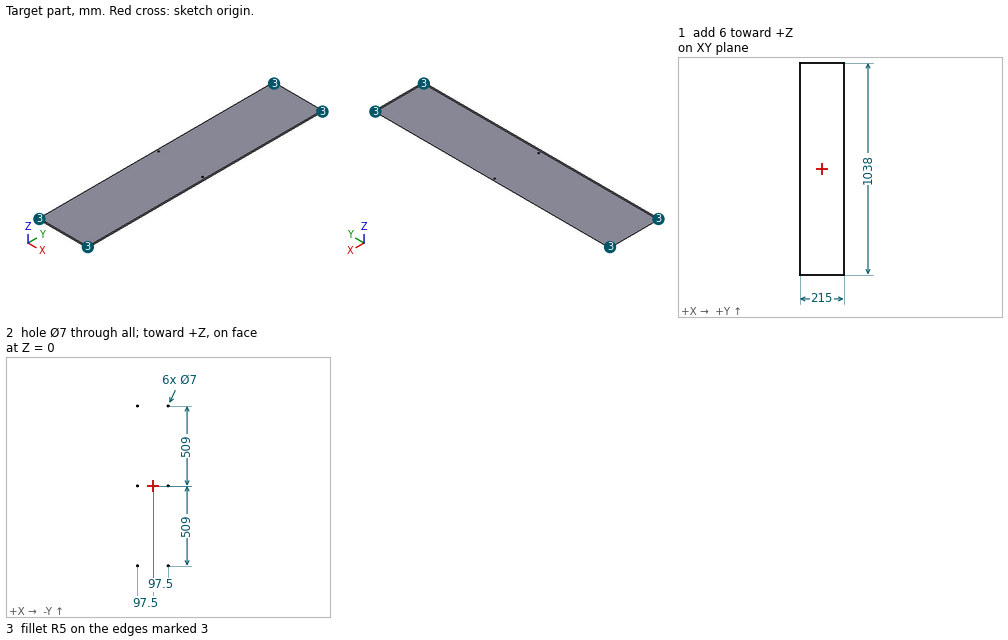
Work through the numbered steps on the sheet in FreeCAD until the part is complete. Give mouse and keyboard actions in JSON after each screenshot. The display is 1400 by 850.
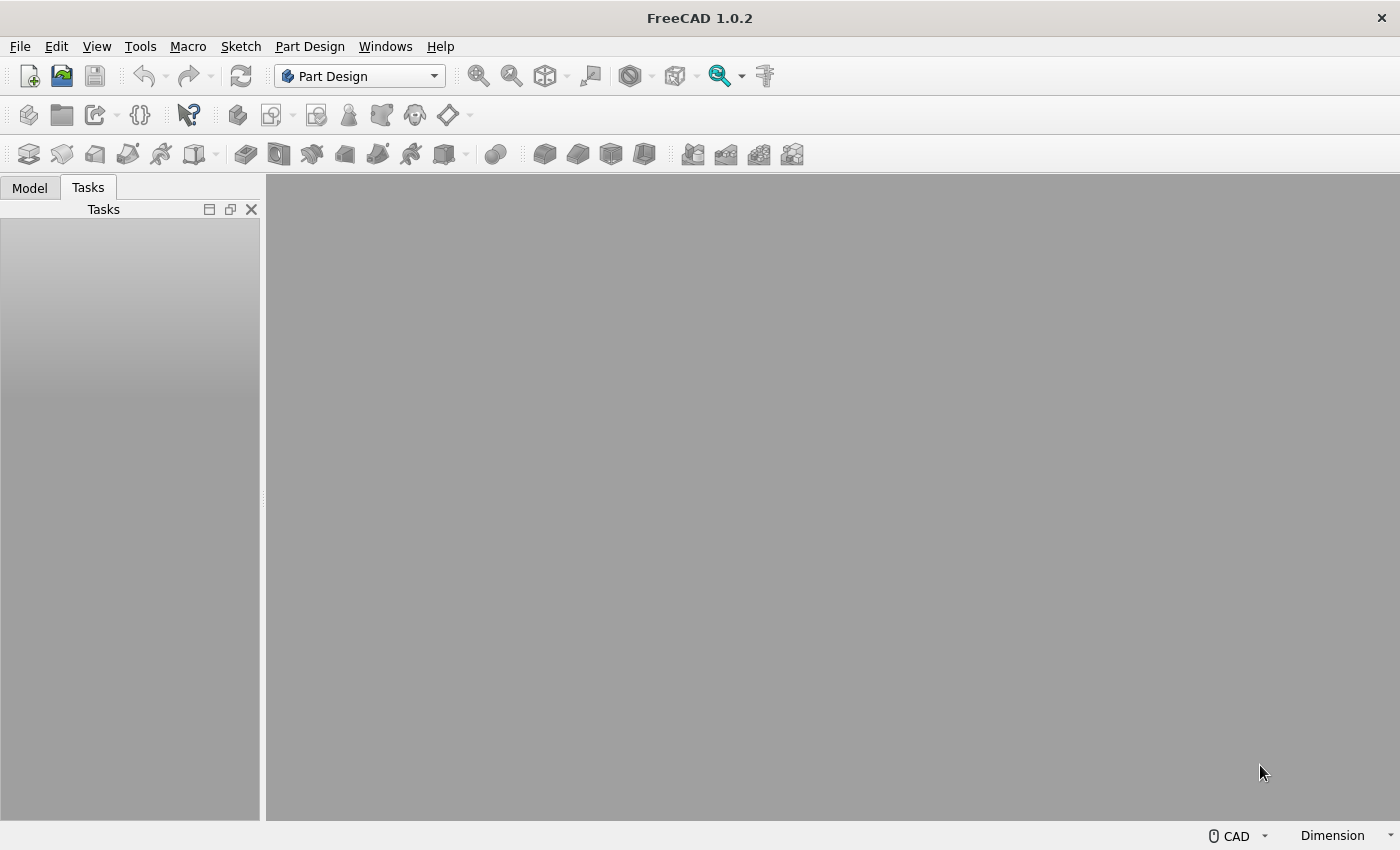
{"action": "left_click", "coordinate": [29, 76]}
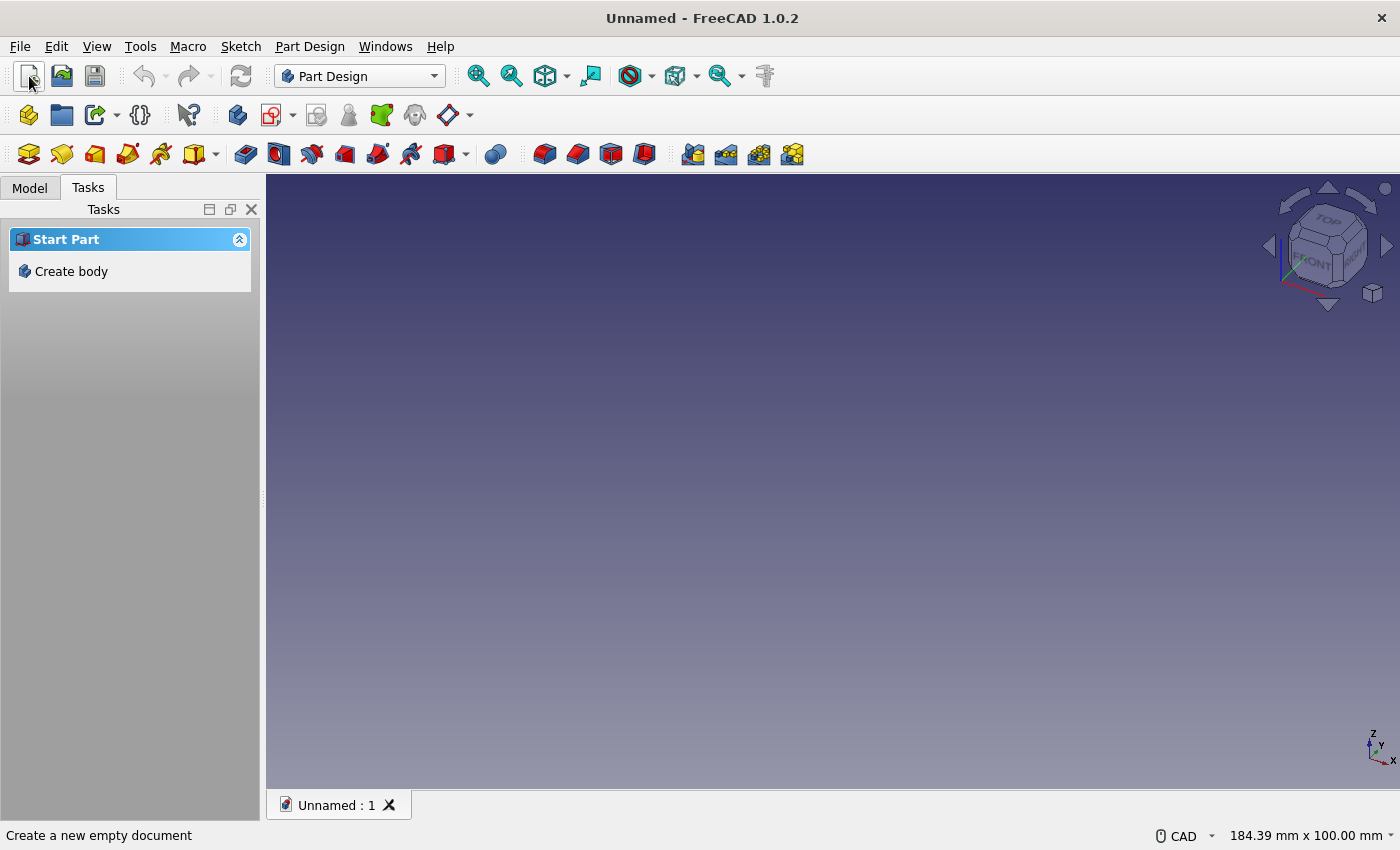
{"action": "left_click", "coordinate": [270, 116]}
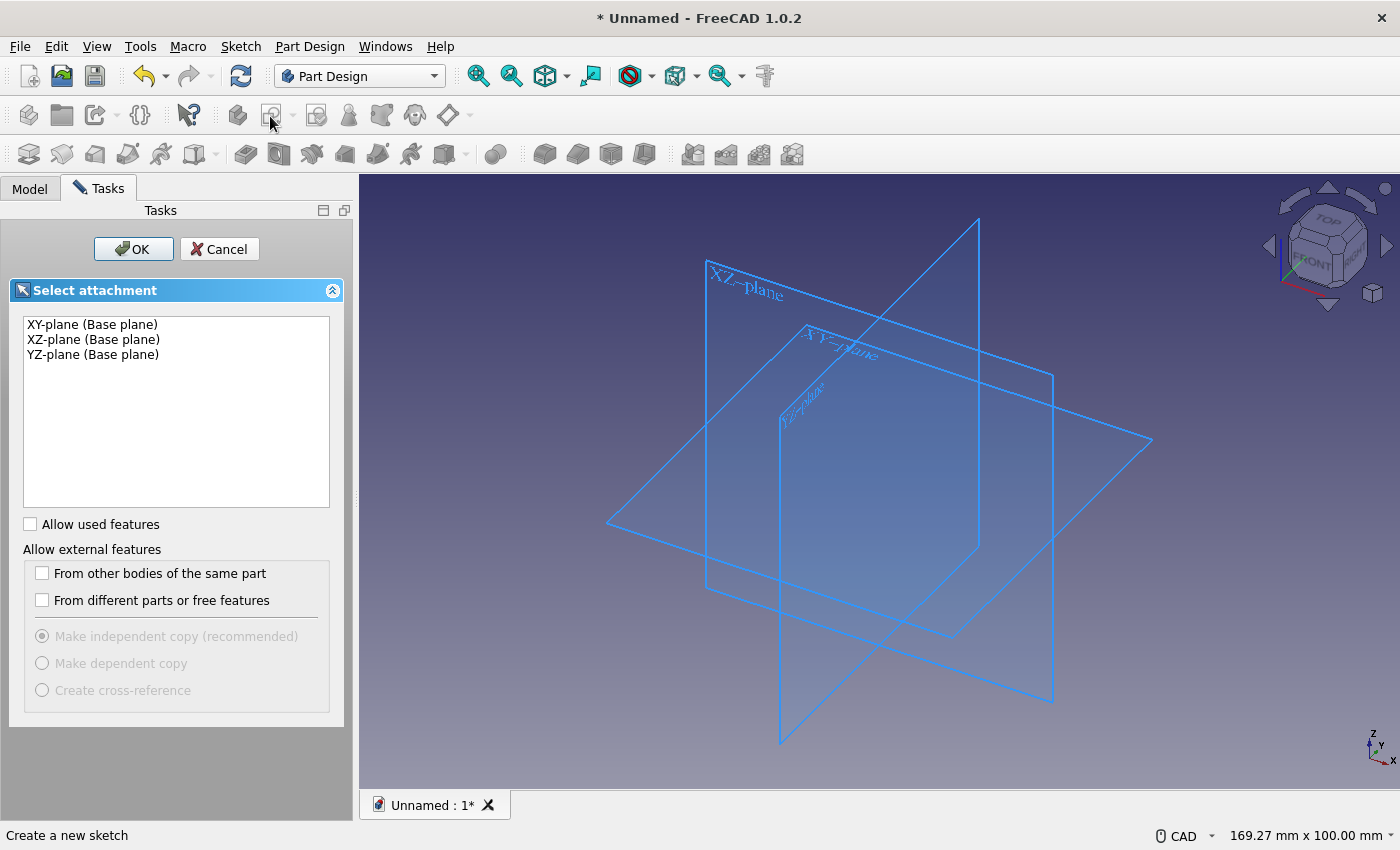
{"action": "left_click", "coordinate": [84, 324]}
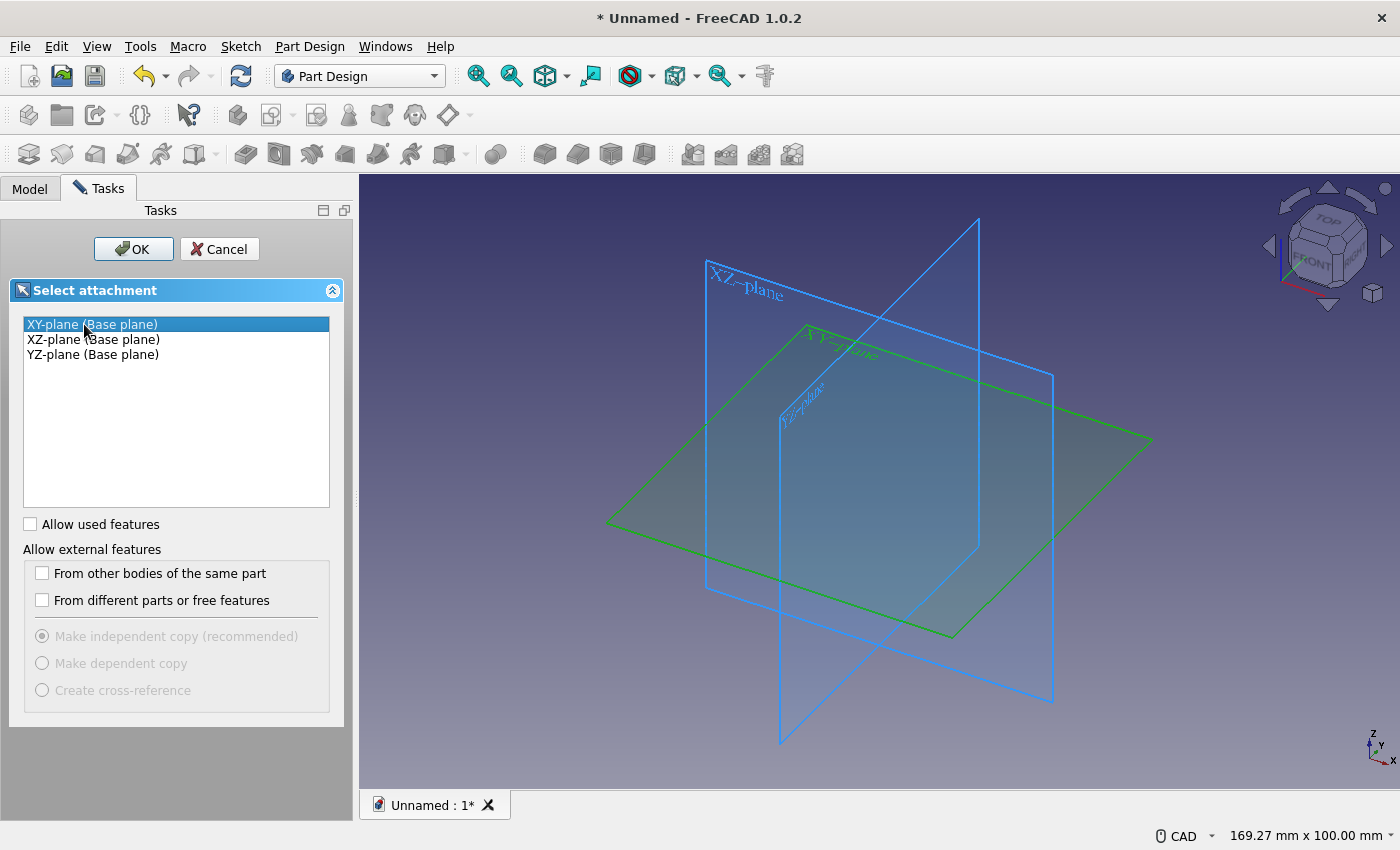
{"action": "left_click", "coordinate": [134, 249]}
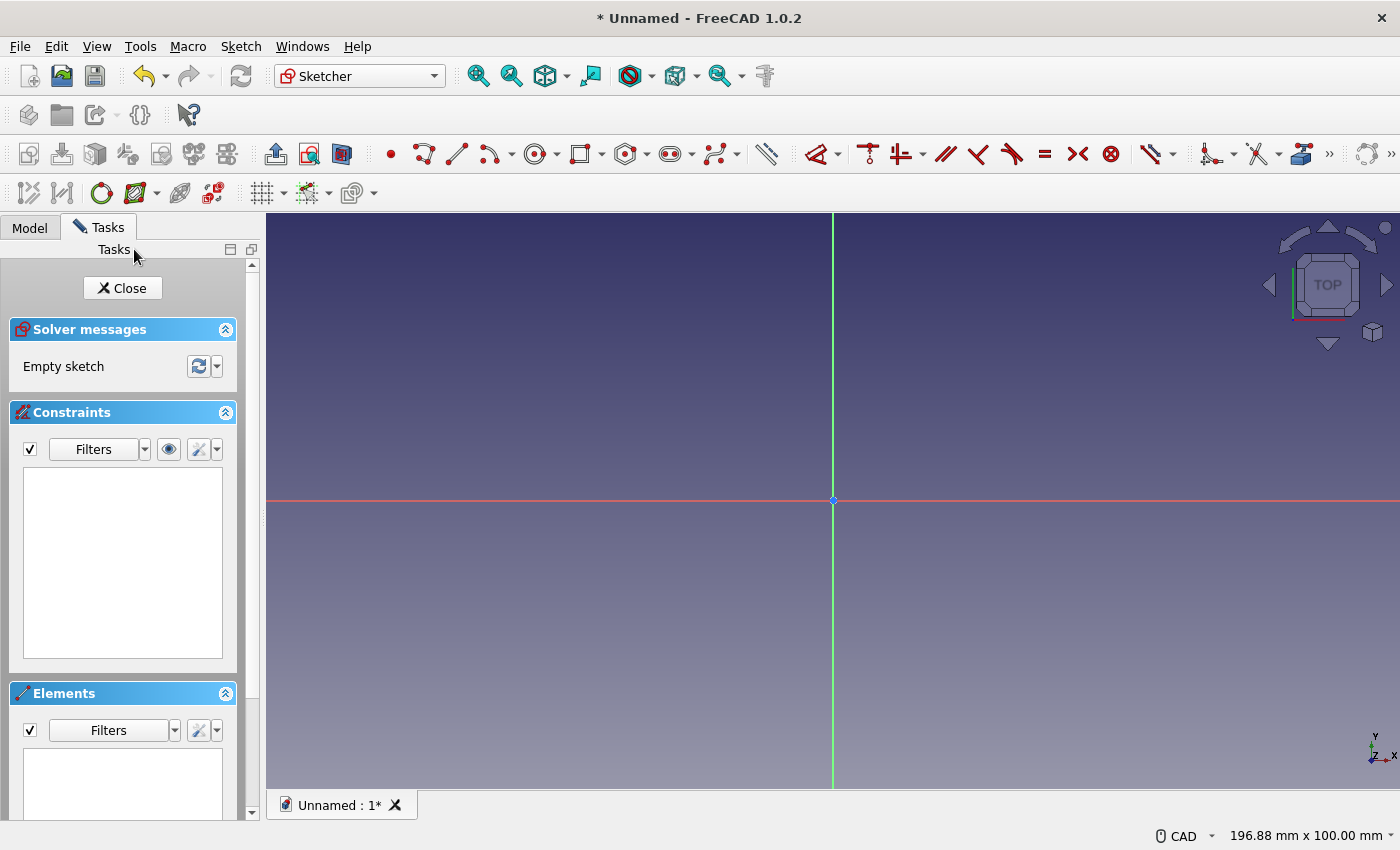
{"action": "scroll", "coordinate": [760, 501], "scroll_direction": "down", "scroll_amount": 14}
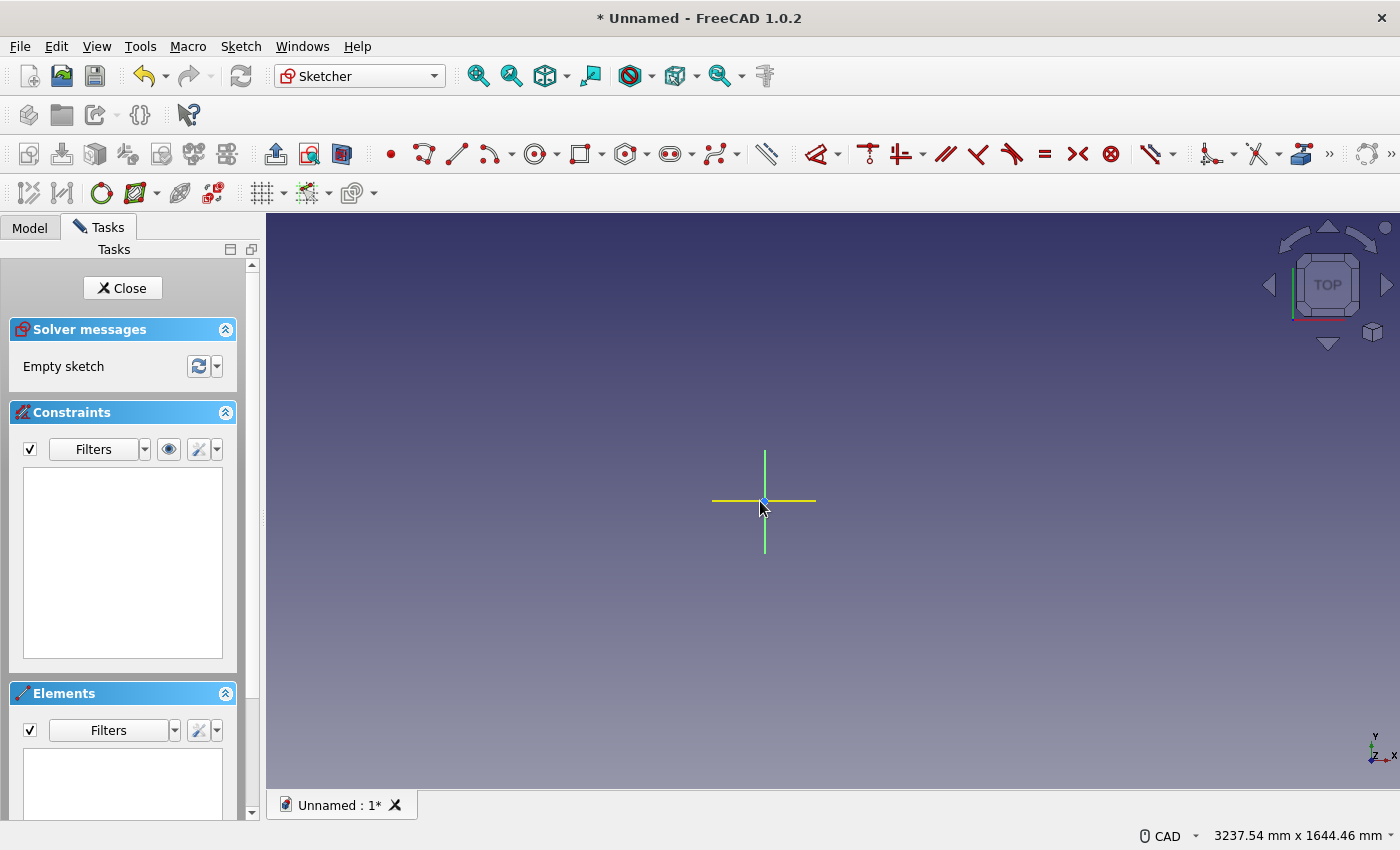
{"action": "key", "text": "g v"}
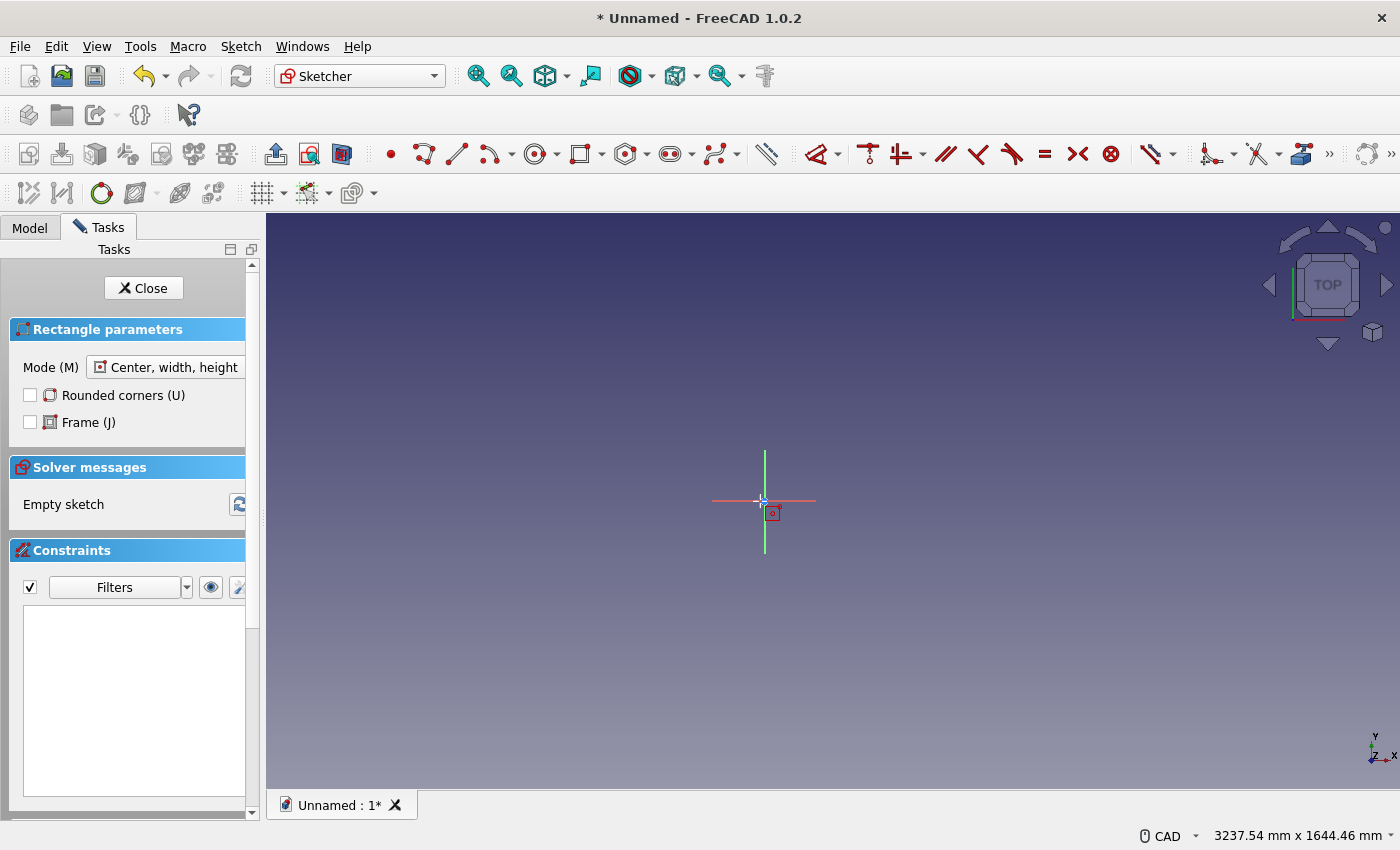
{"action": "left_click", "coordinate": [765, 501]}
{"action": "left_click", "coordinate": [803, 320]}
{"action": "key", "text": "Escape"}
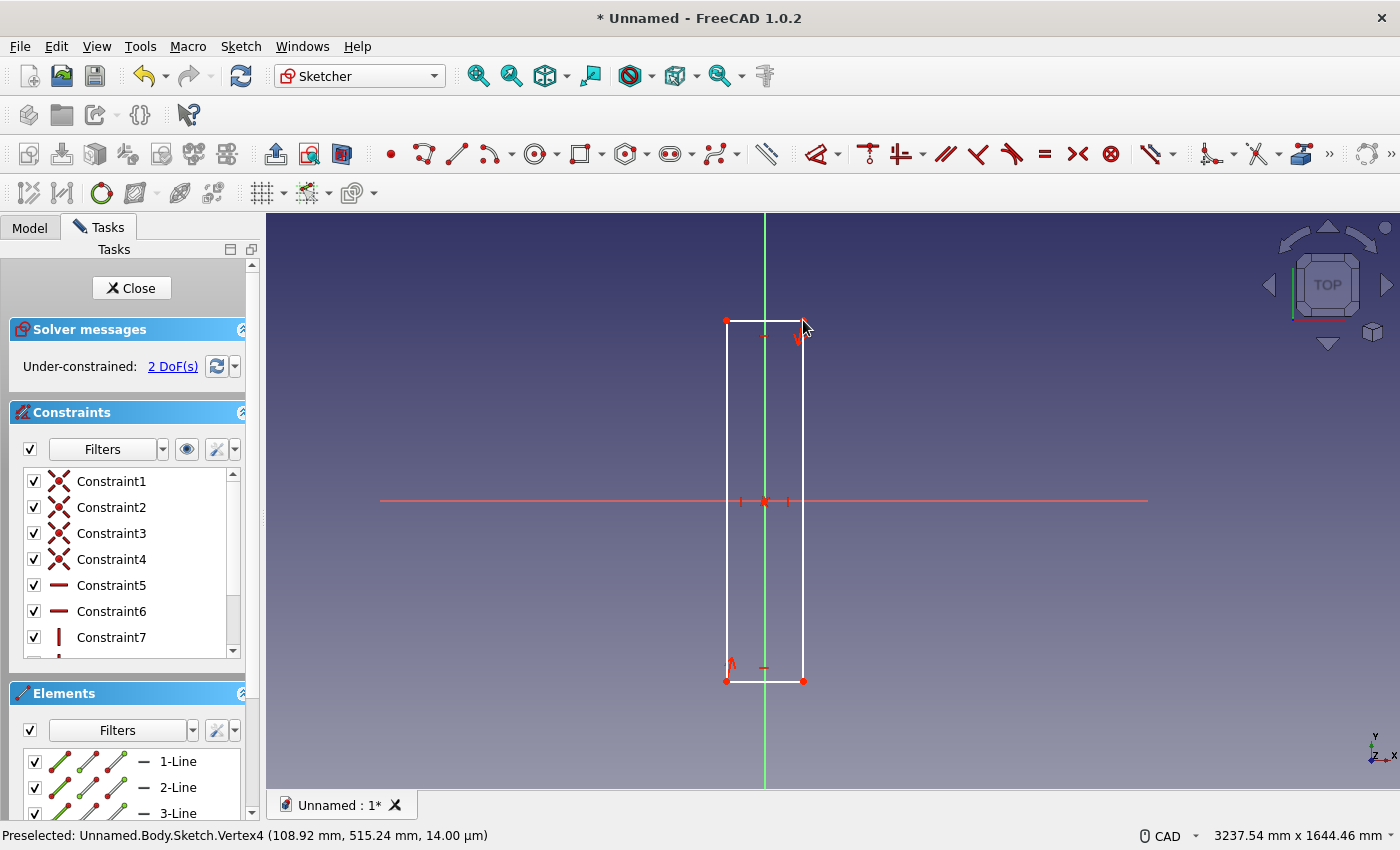
{"action": "left_click", "coordinate": [750, 682]}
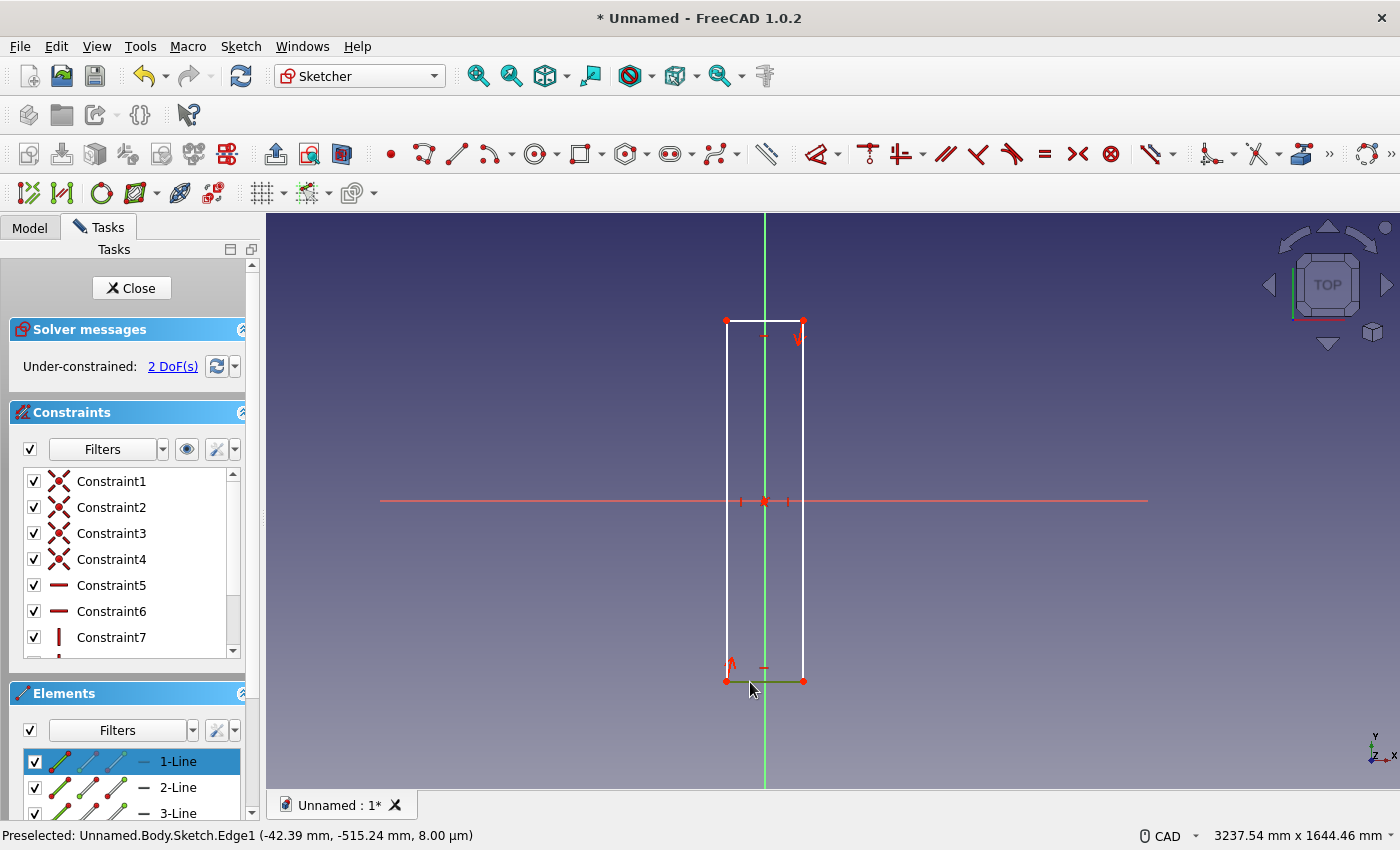
{"action": "key", "text": "l"}